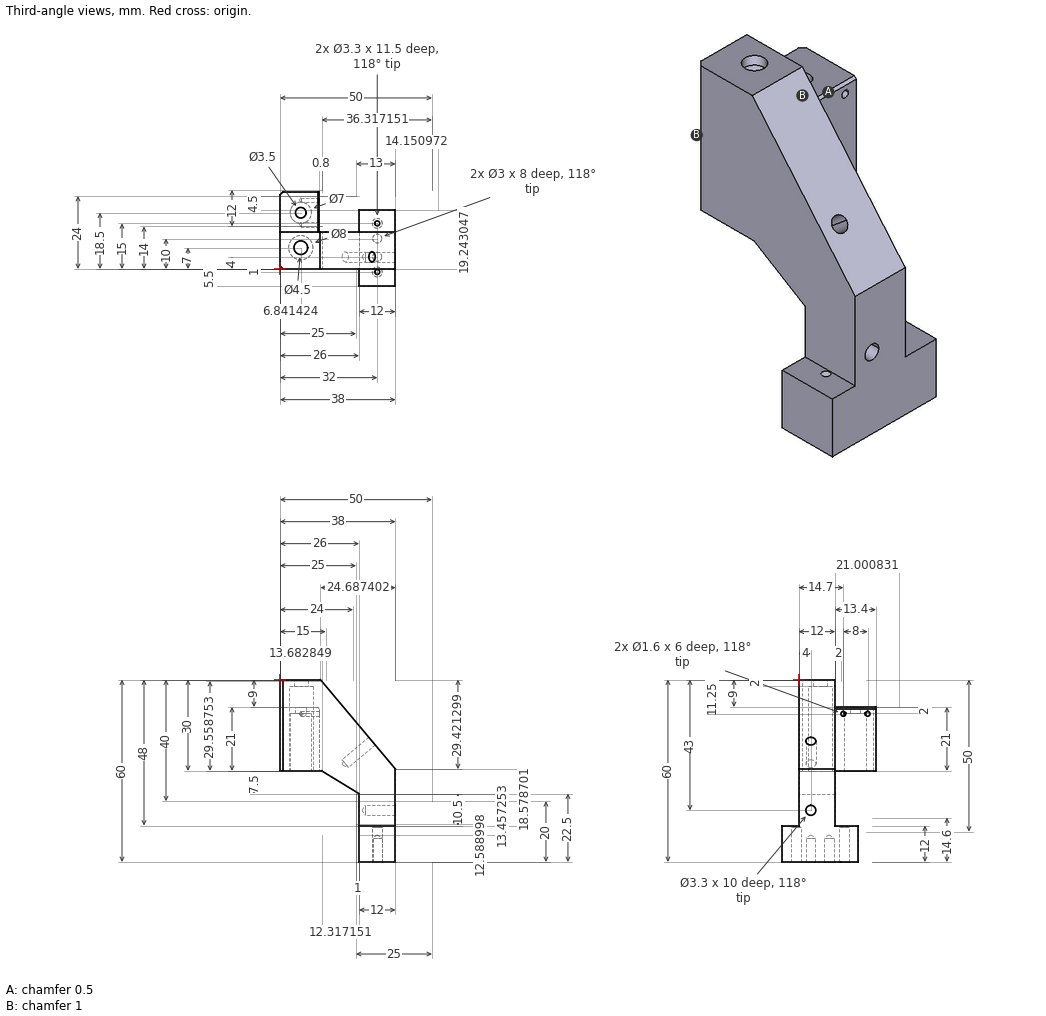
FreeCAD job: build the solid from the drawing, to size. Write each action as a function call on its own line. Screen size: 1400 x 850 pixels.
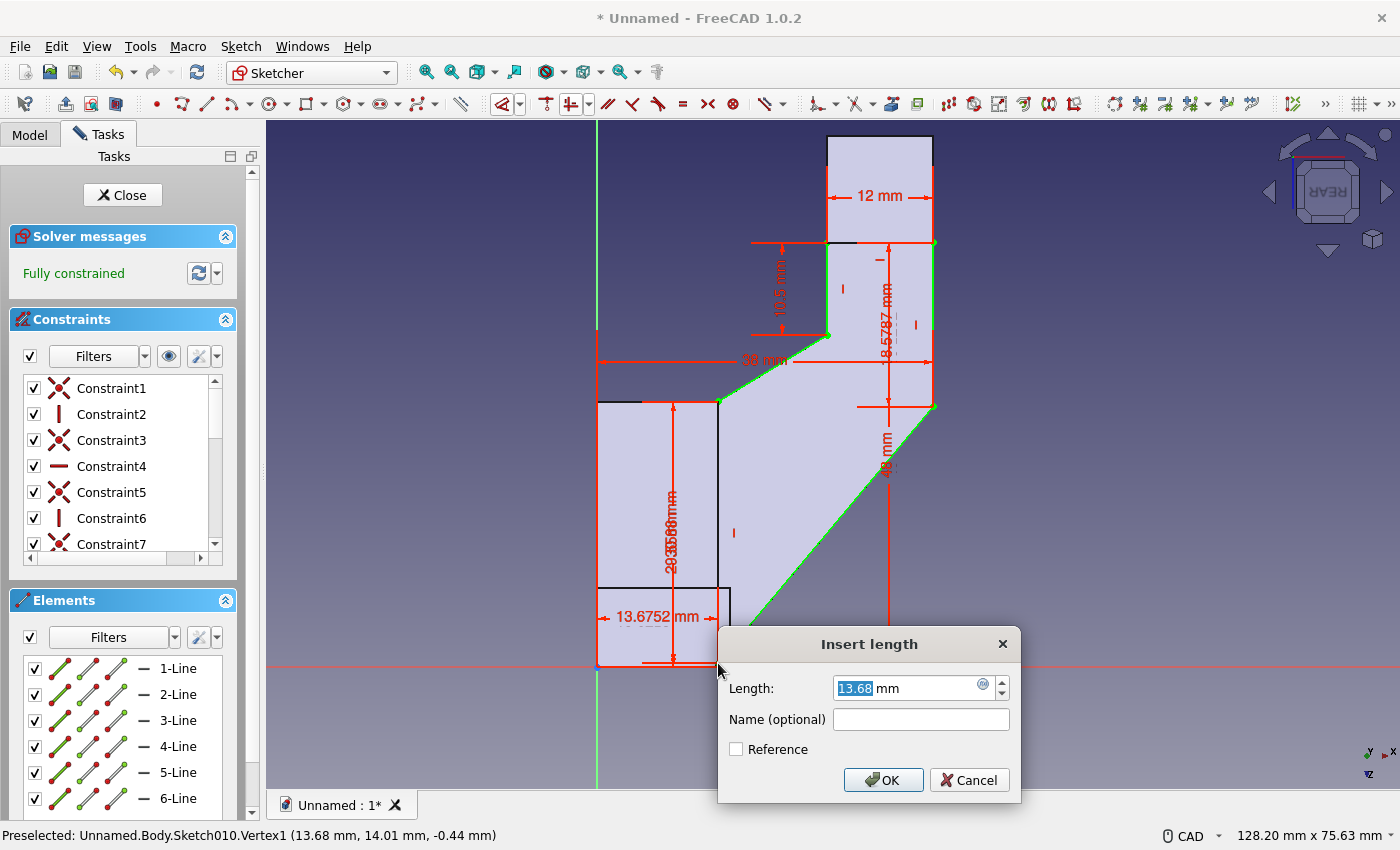
text(13.682849)
key(Return)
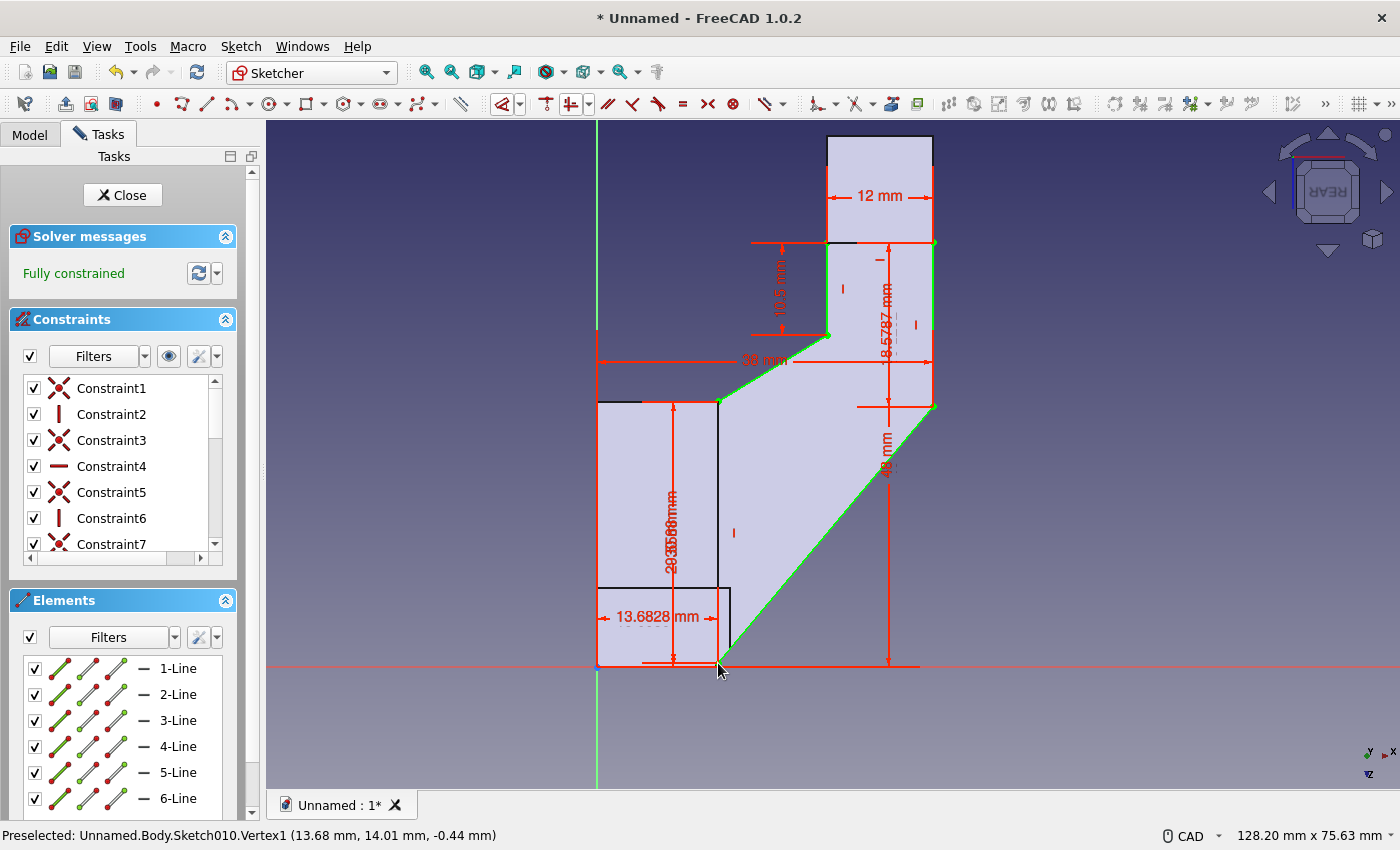
click(123, 195)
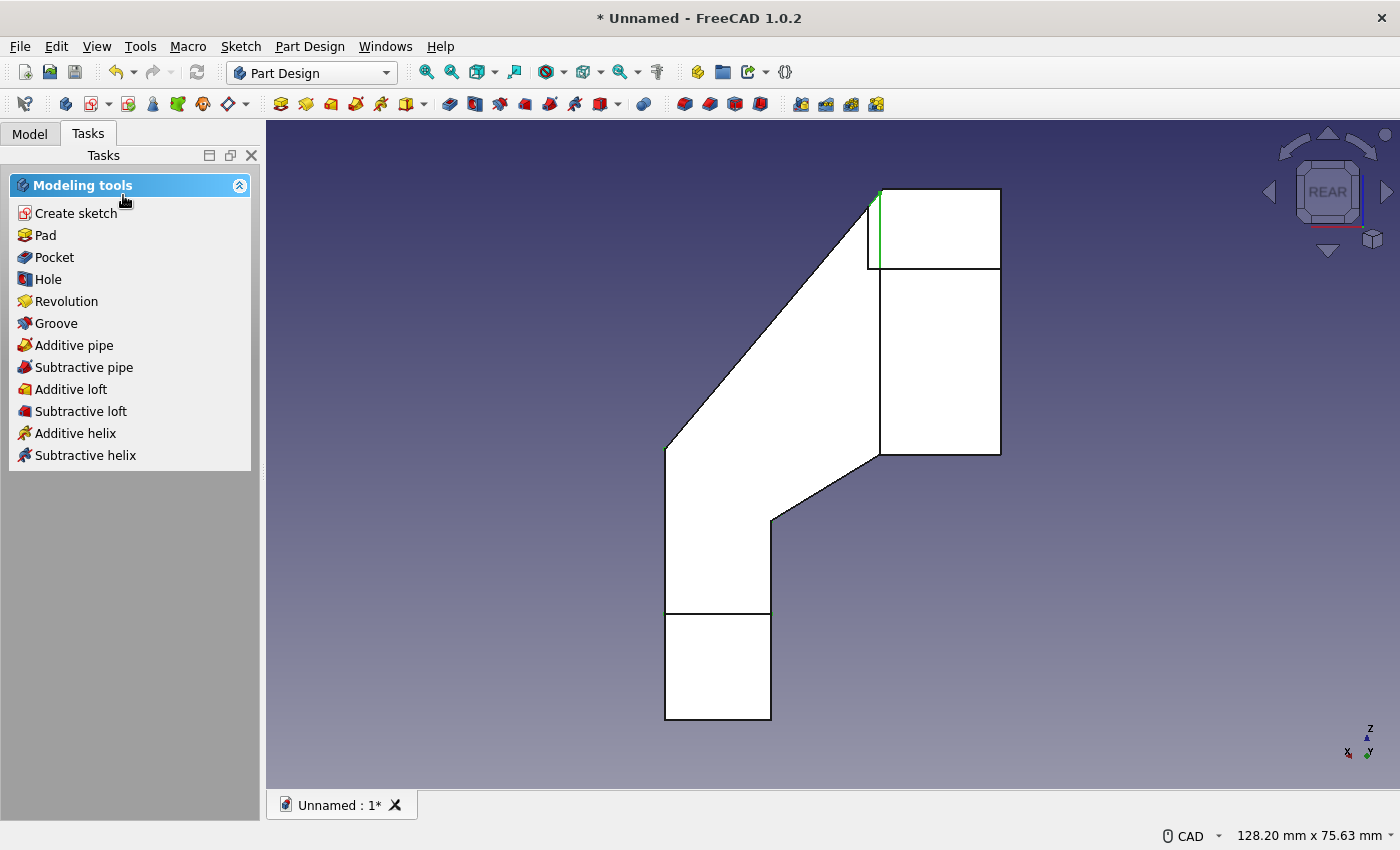
click(450, 104)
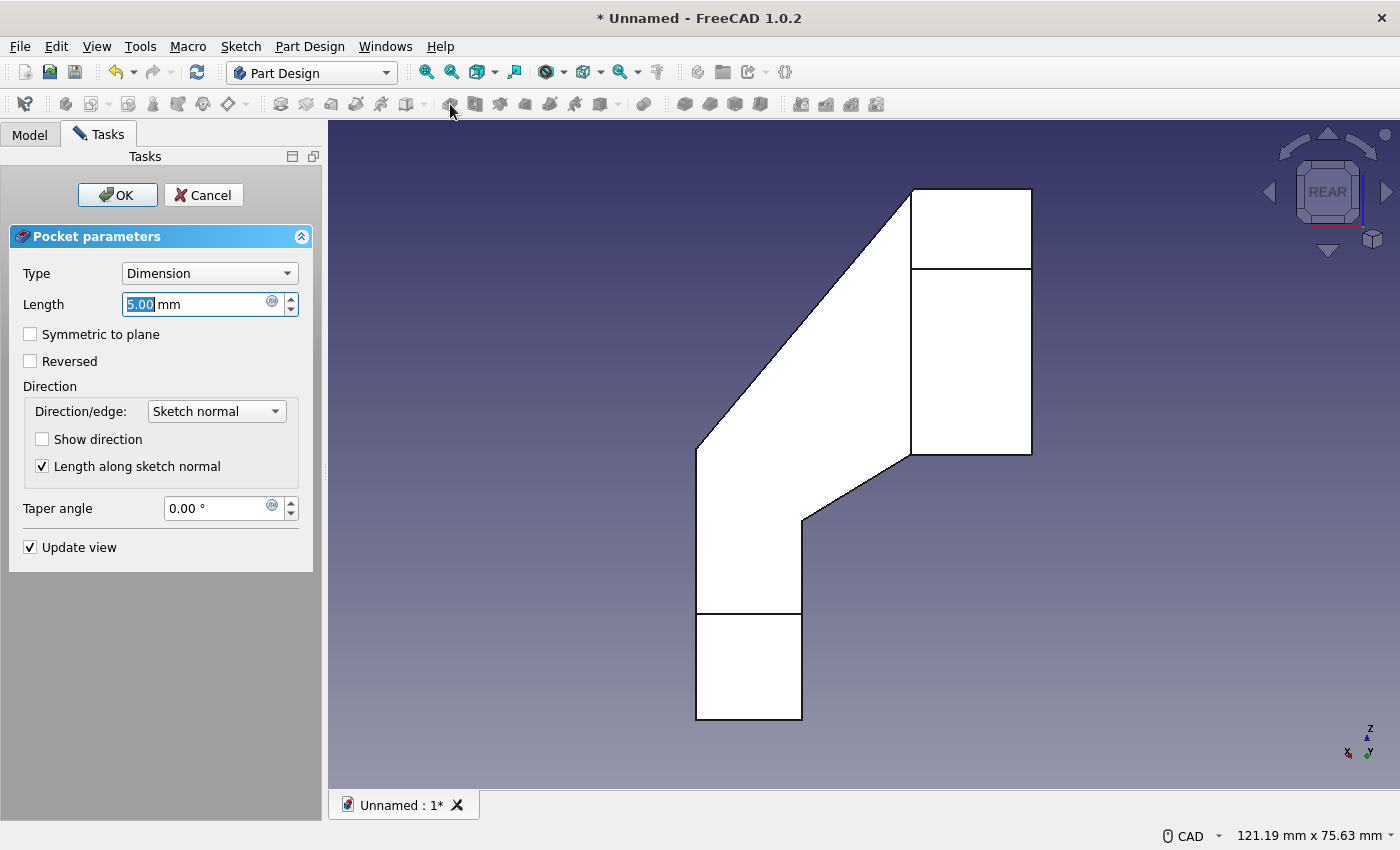
text(2)
key(Tab)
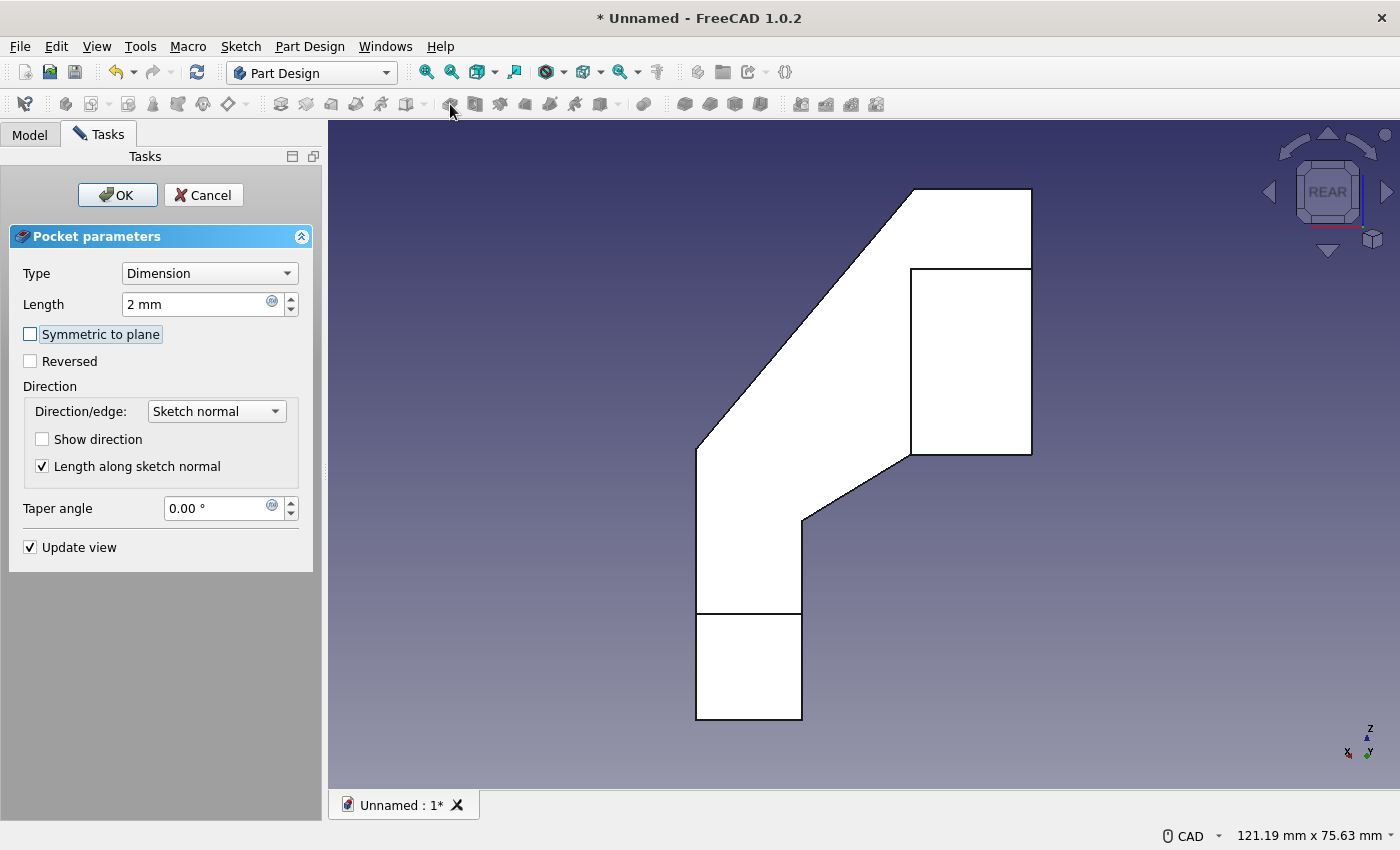
click(118, 195)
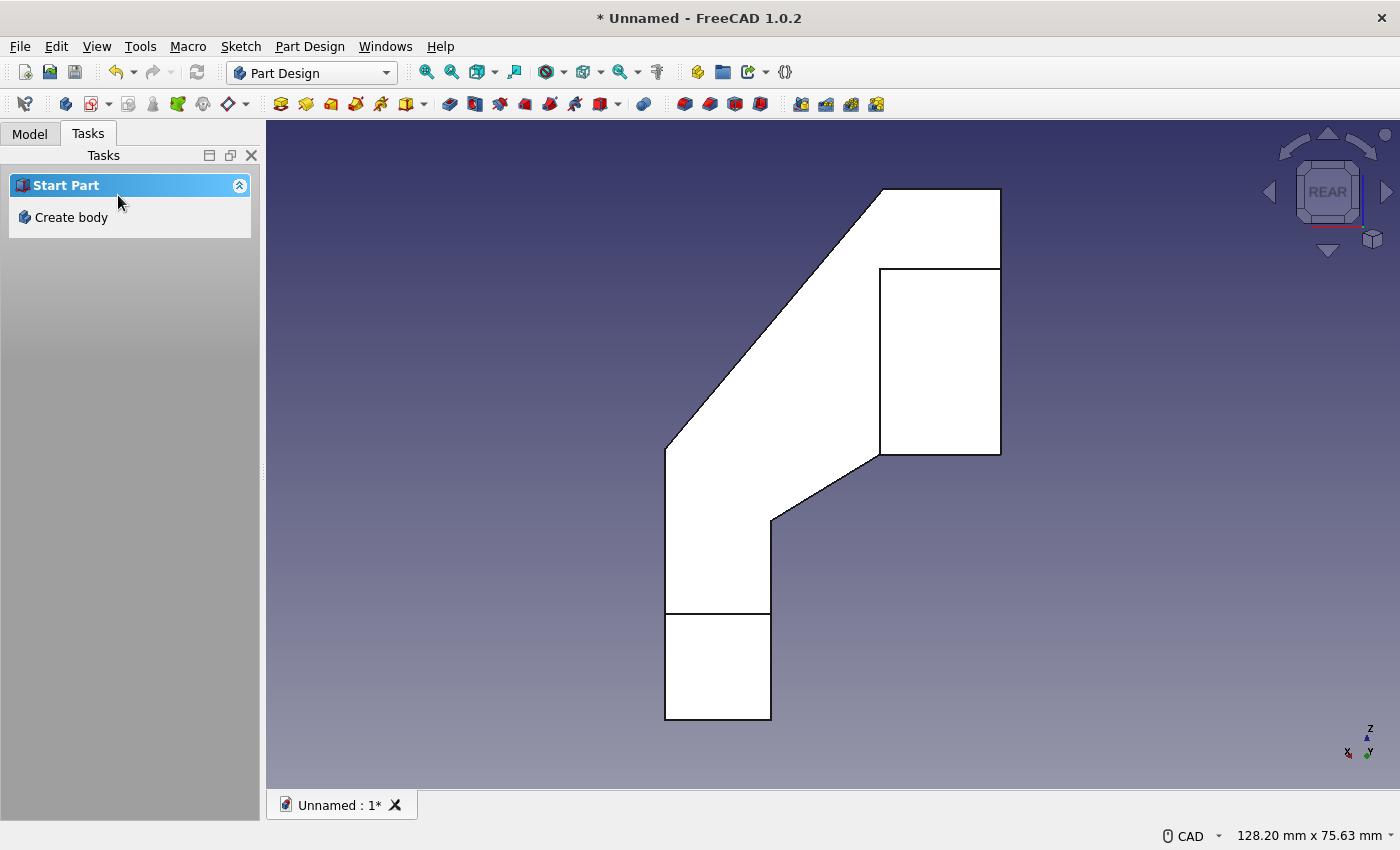
key(5)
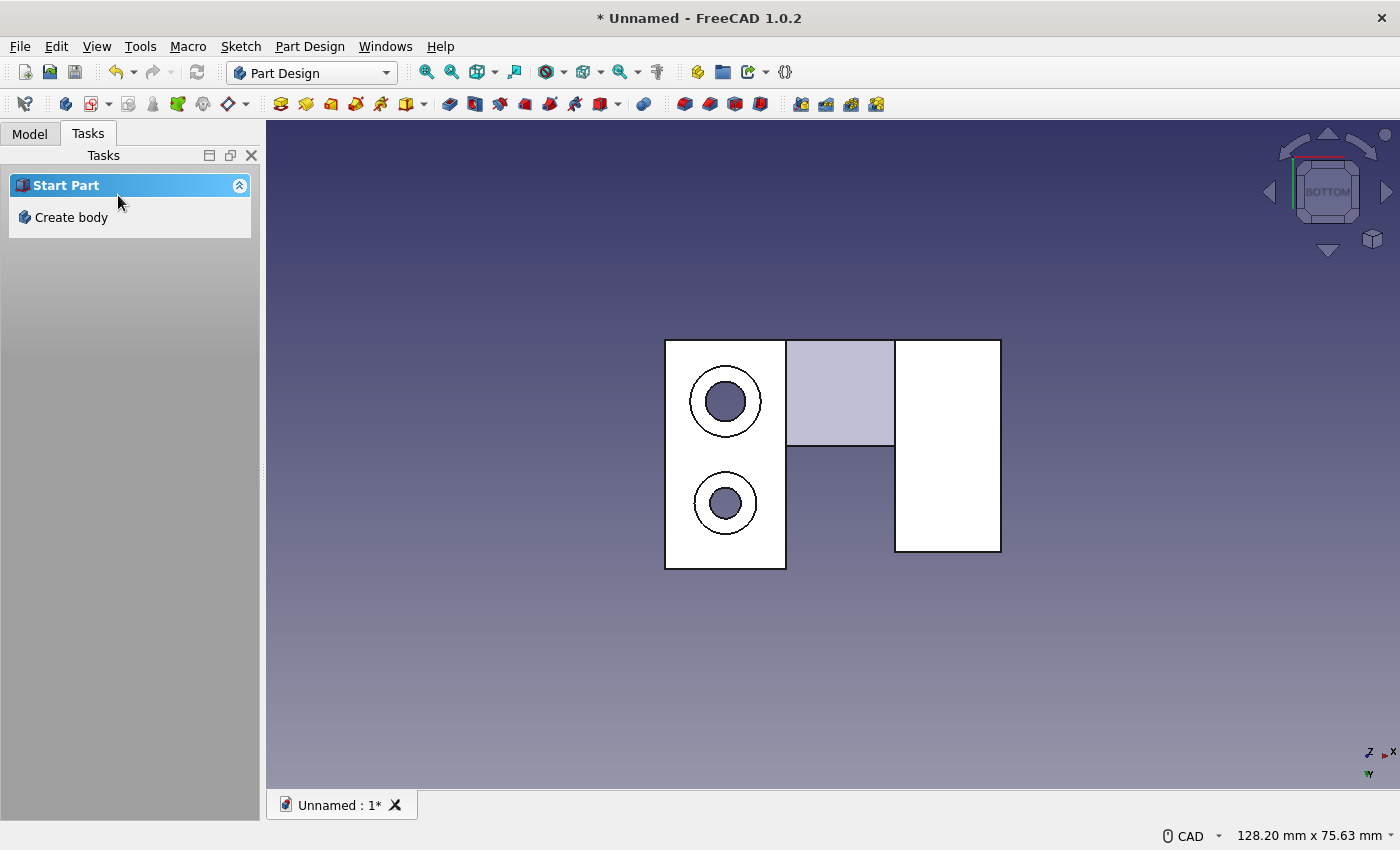
click(427, 72)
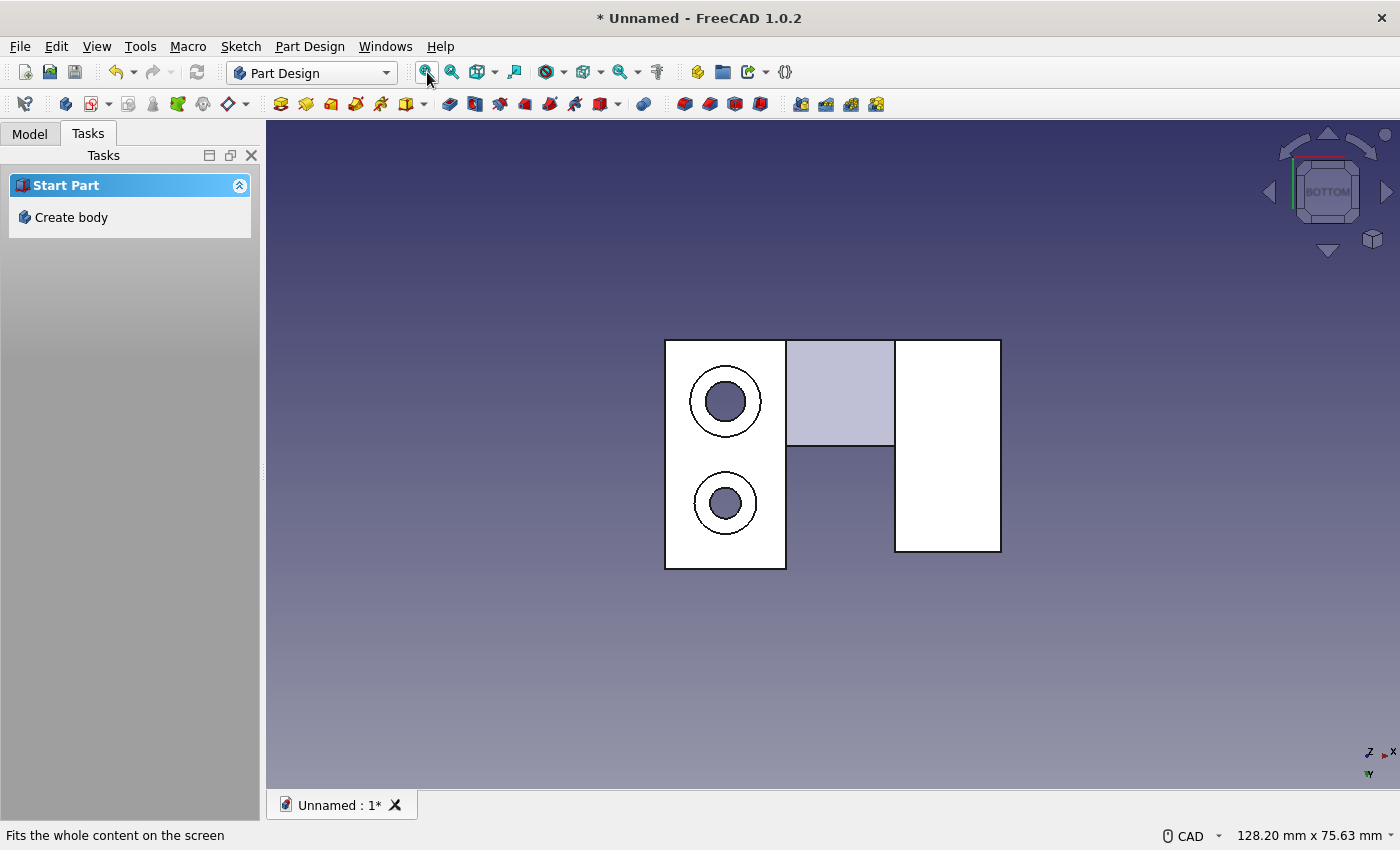
click(948, 475)